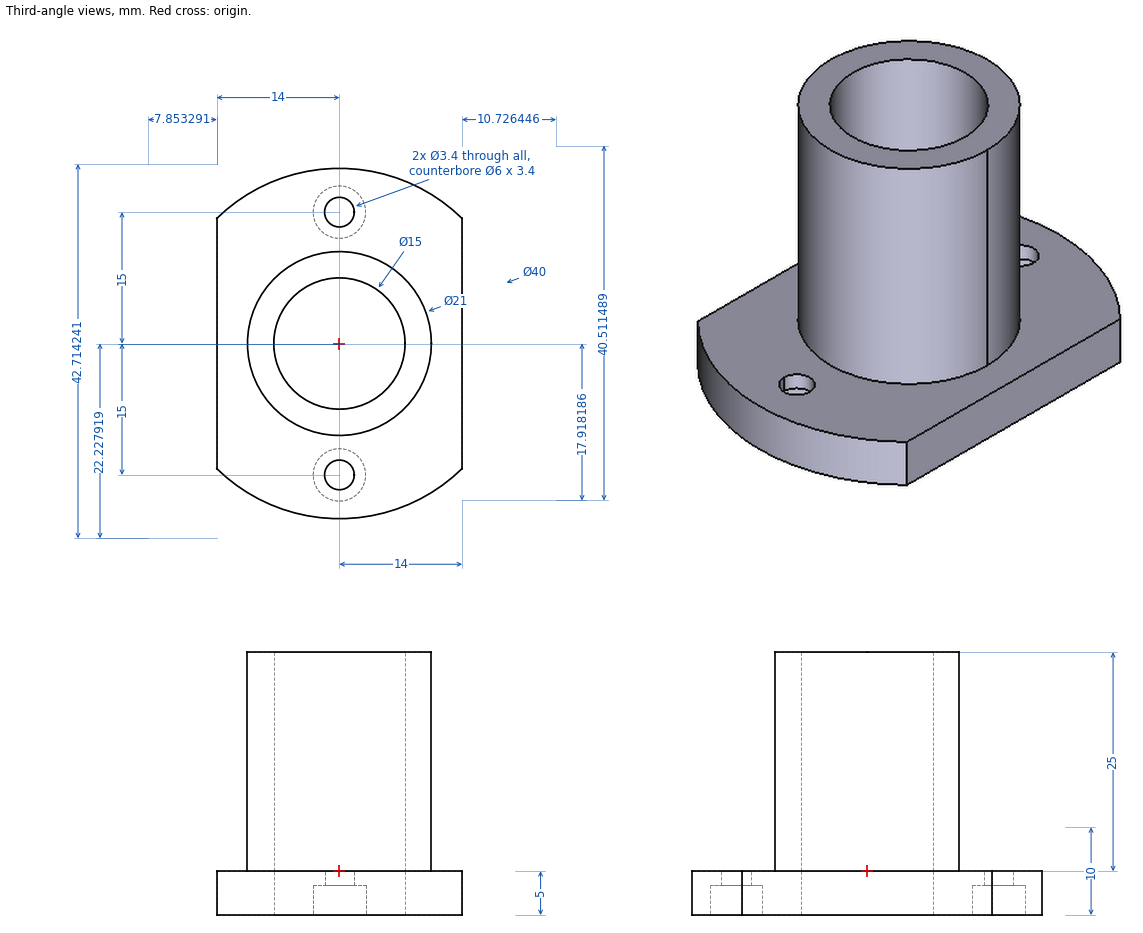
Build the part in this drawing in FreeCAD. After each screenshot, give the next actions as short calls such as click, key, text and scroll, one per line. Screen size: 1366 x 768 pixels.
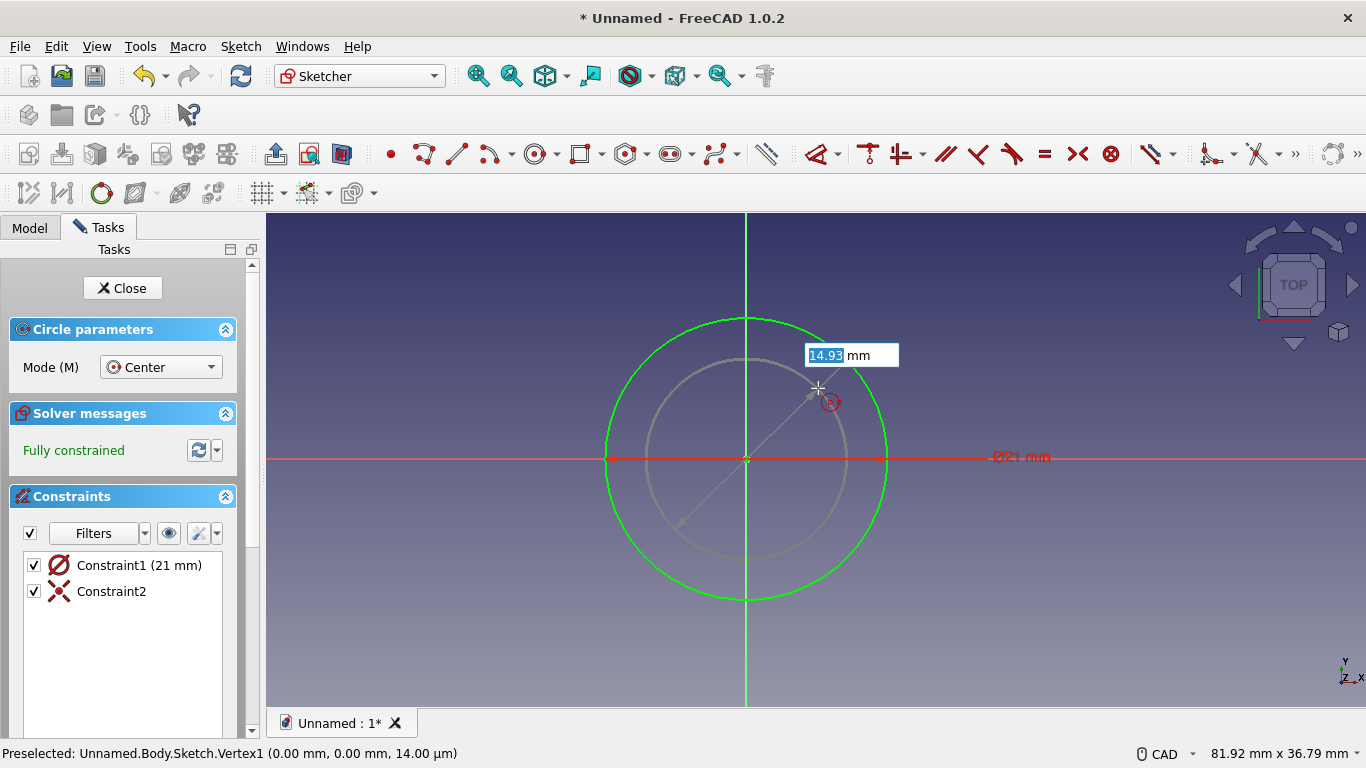
text(15)
key(Return)
key(Escape)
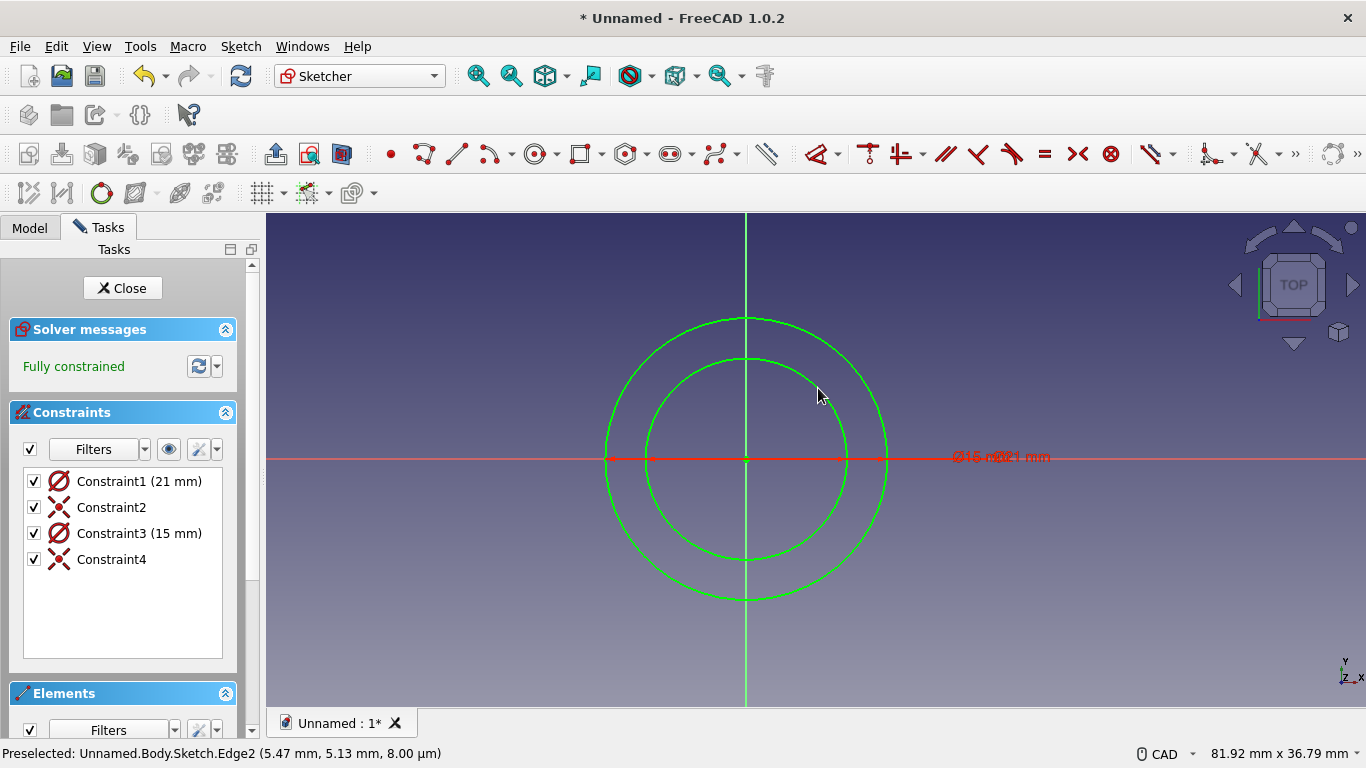
click(123, 288)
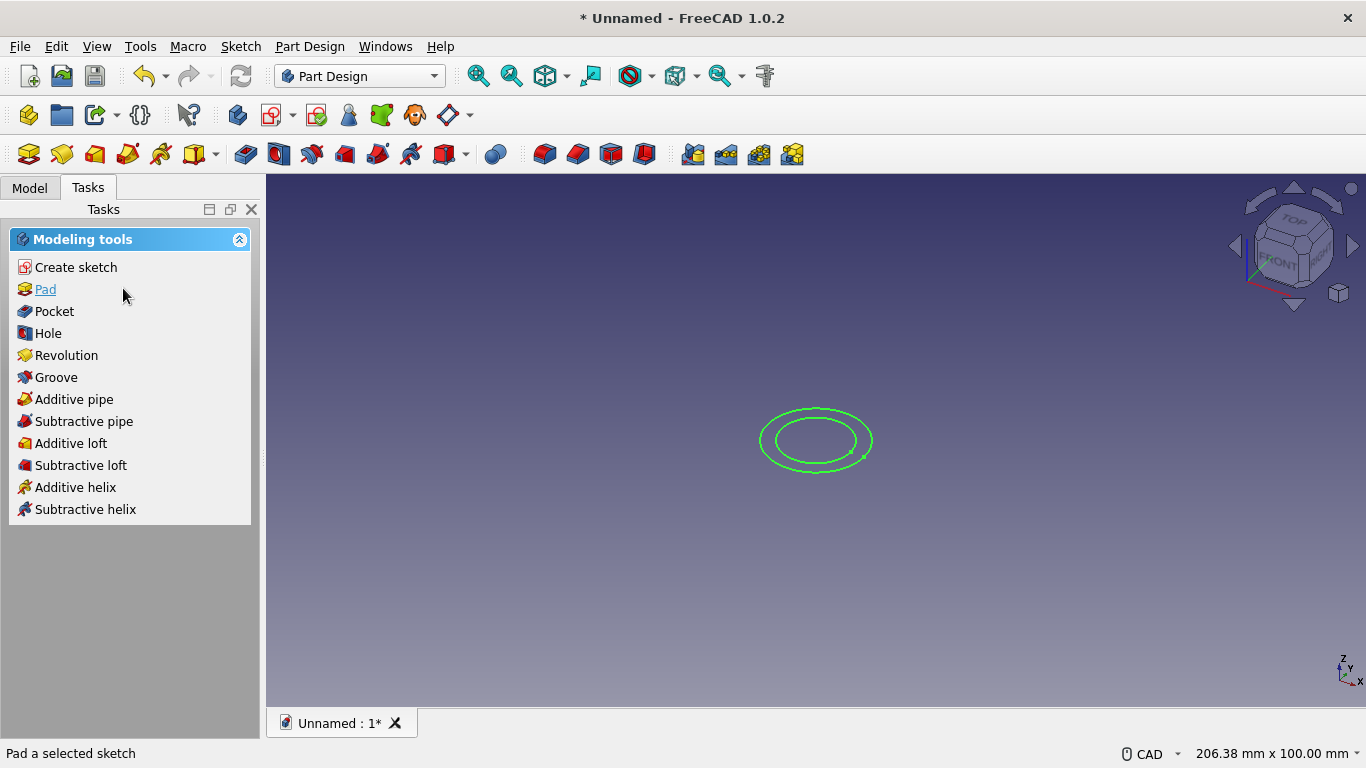
click(29, 154)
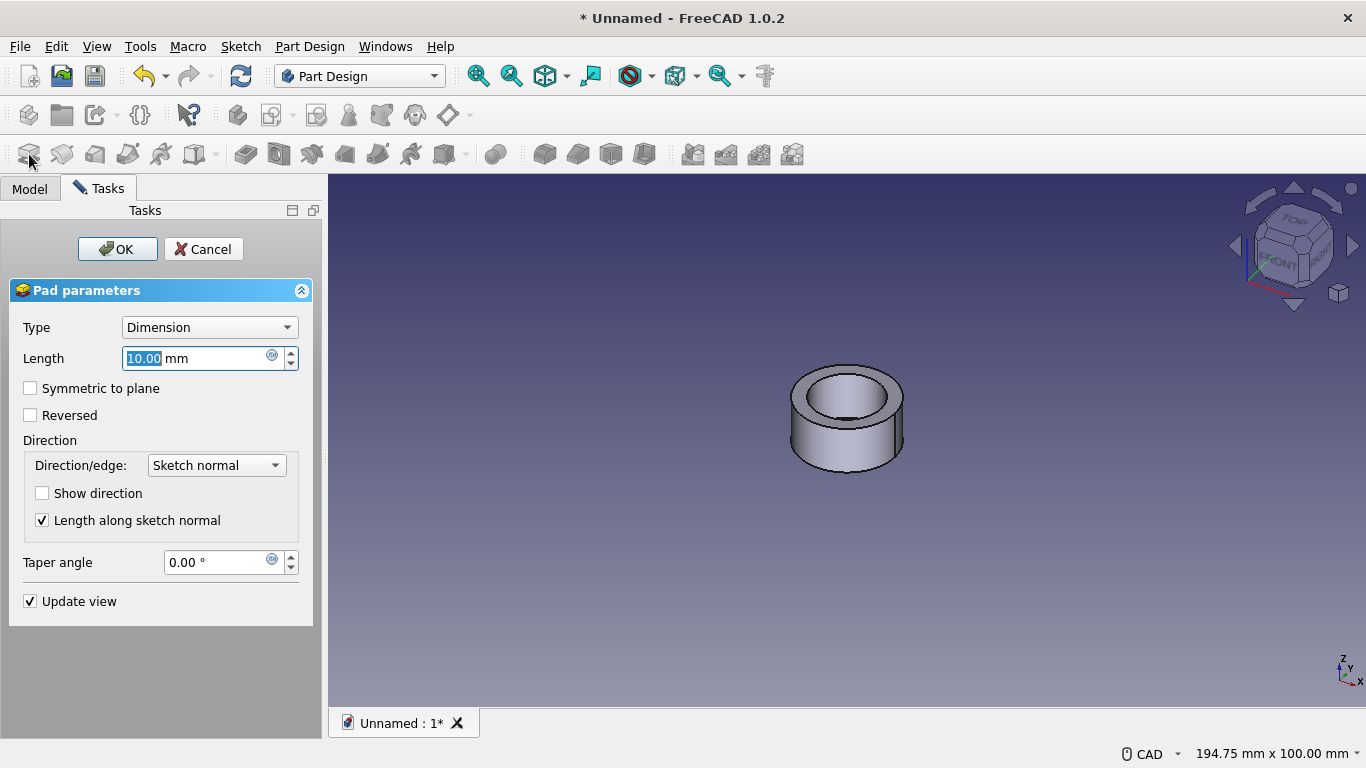
text(25)
key(Tab)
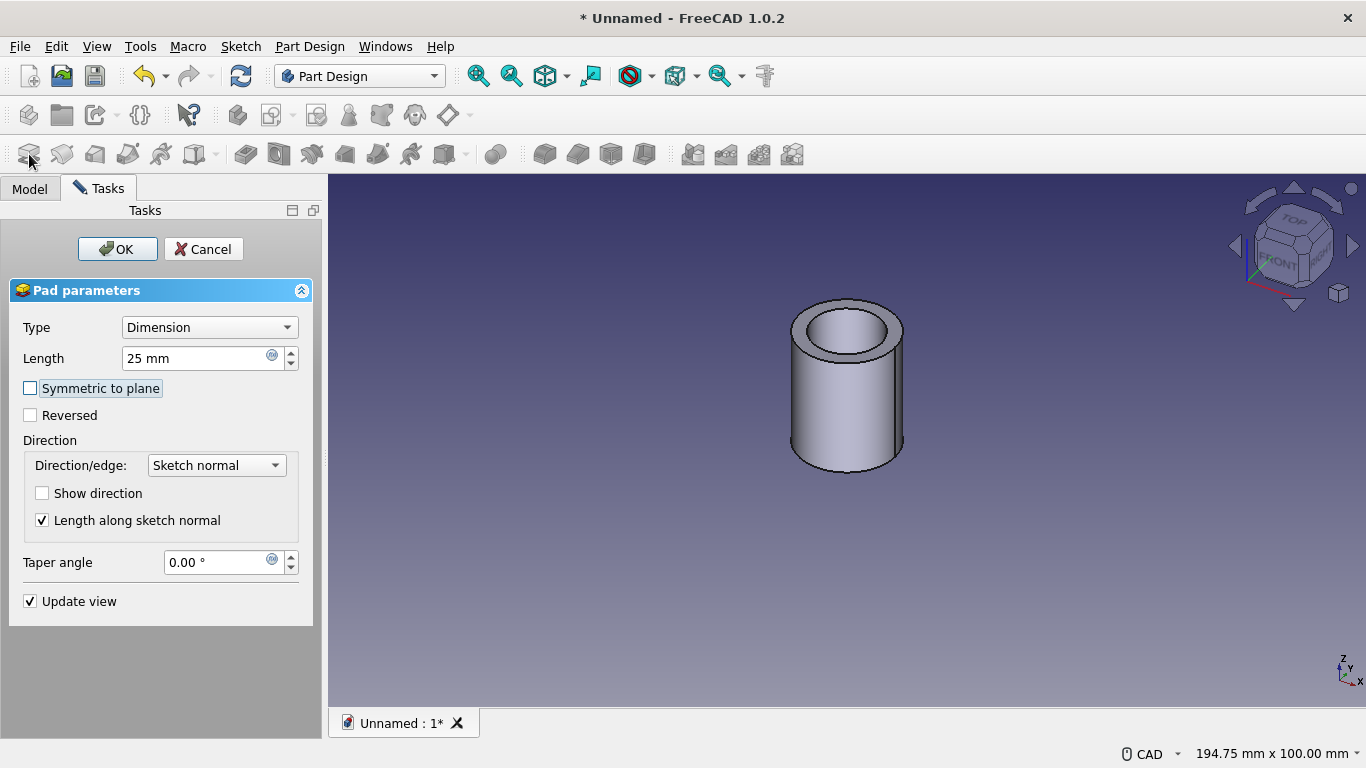
click(118, 249)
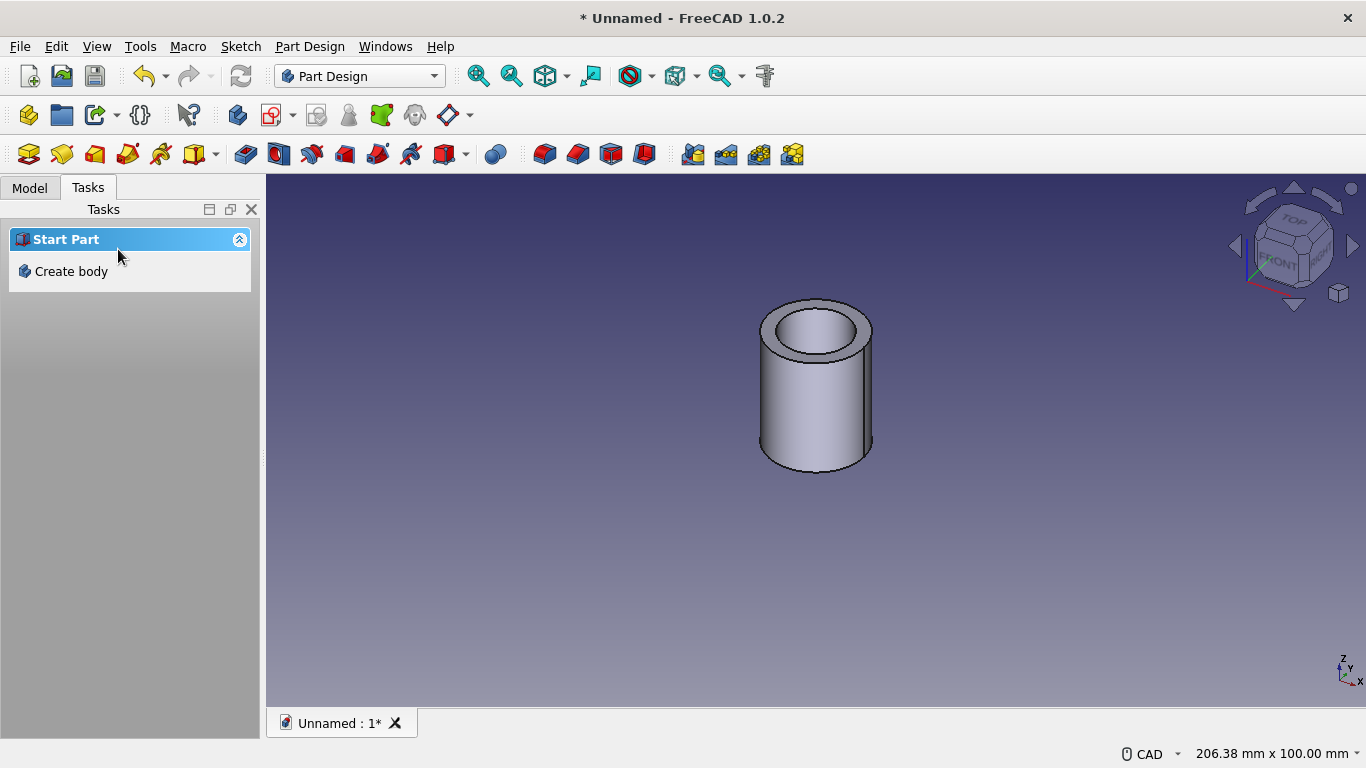
click(479, 76)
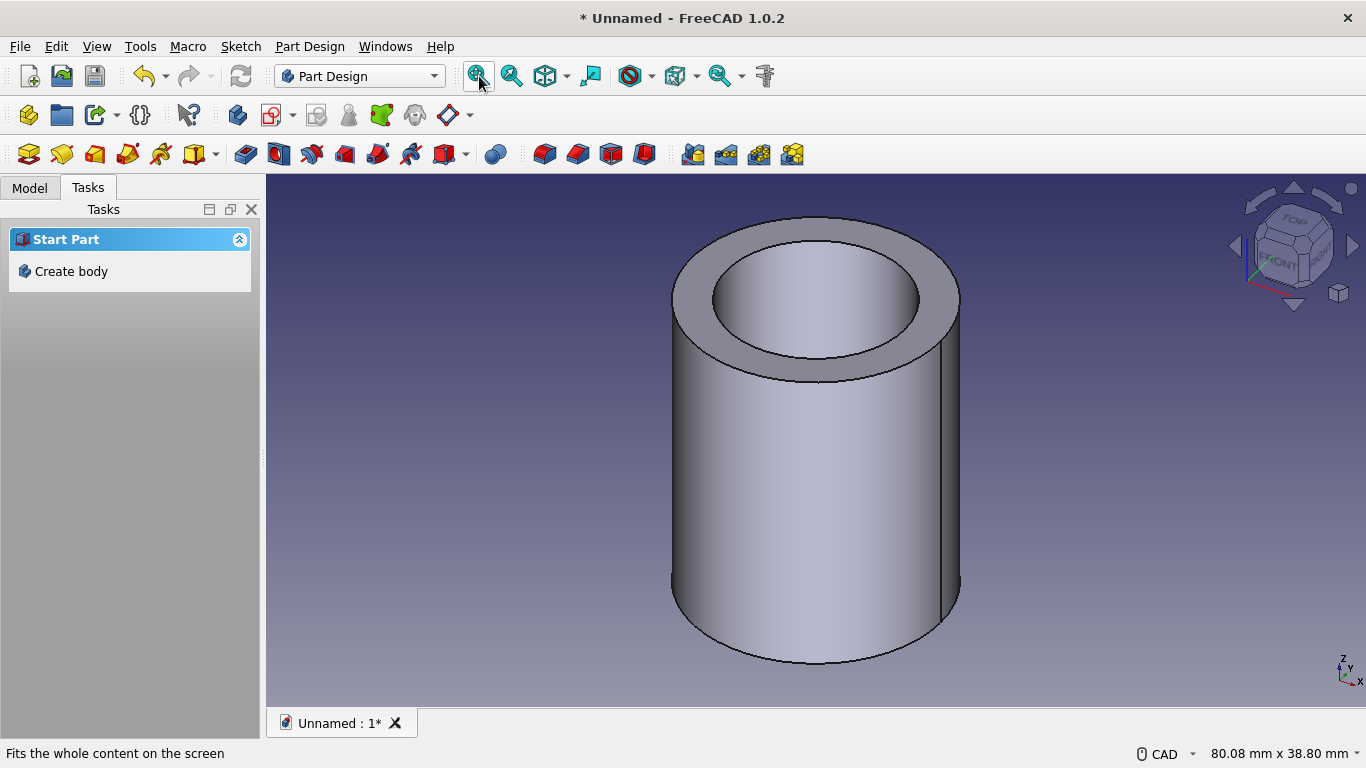
click(30, 188)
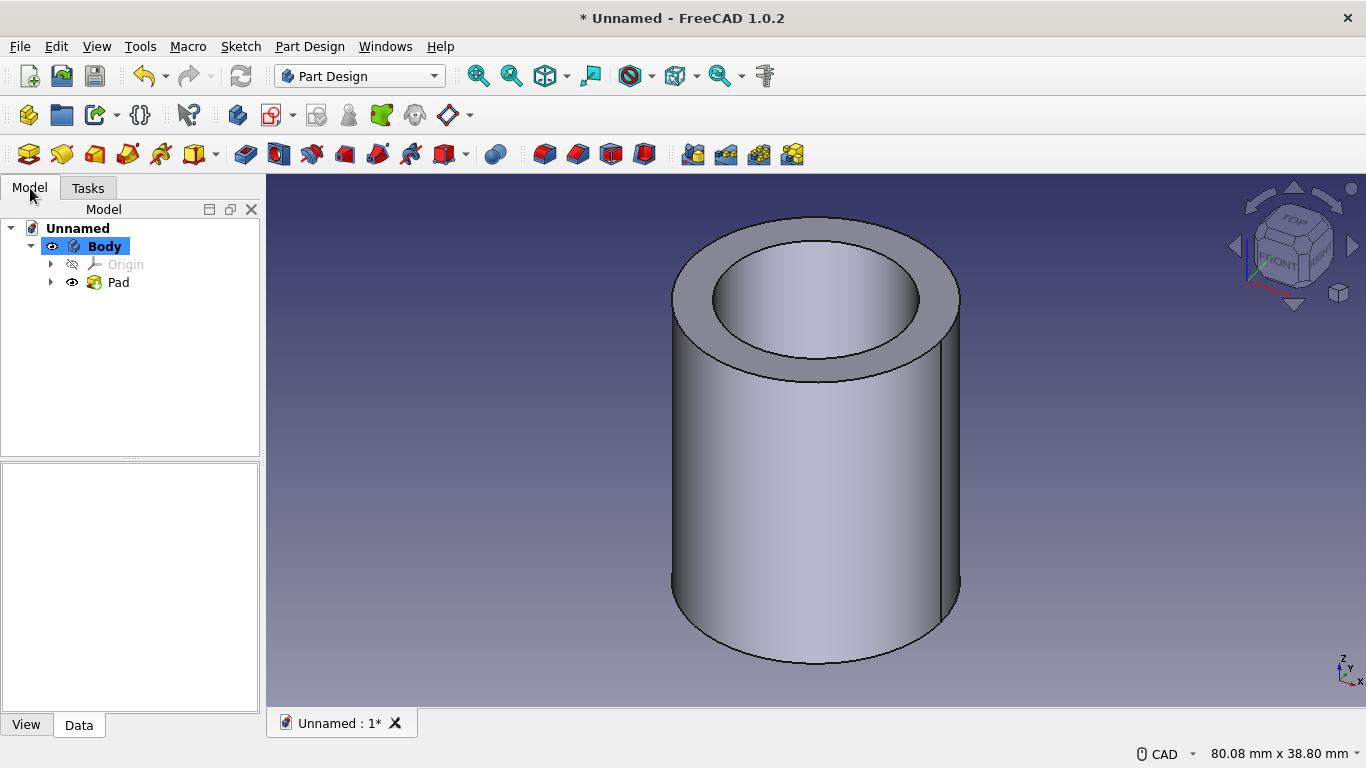
click(51, 264)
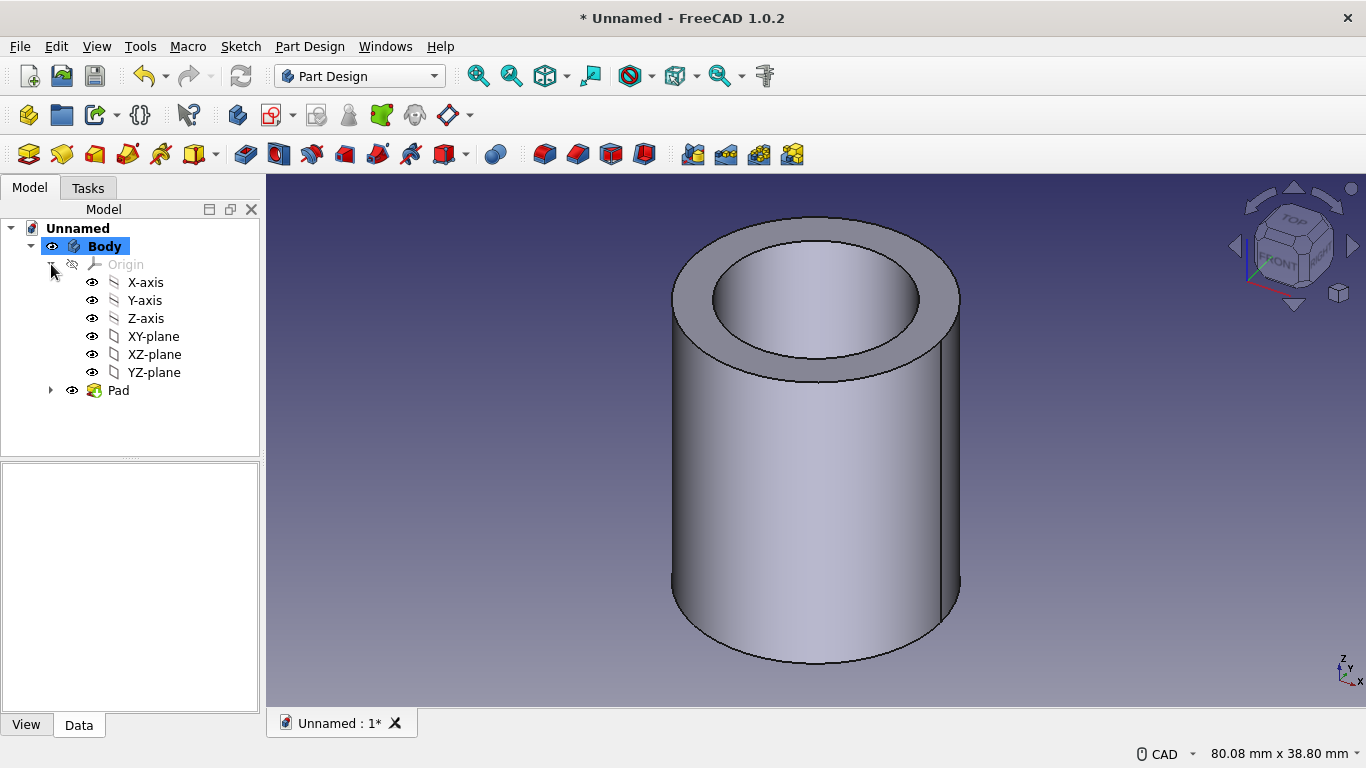
click(137, 336)